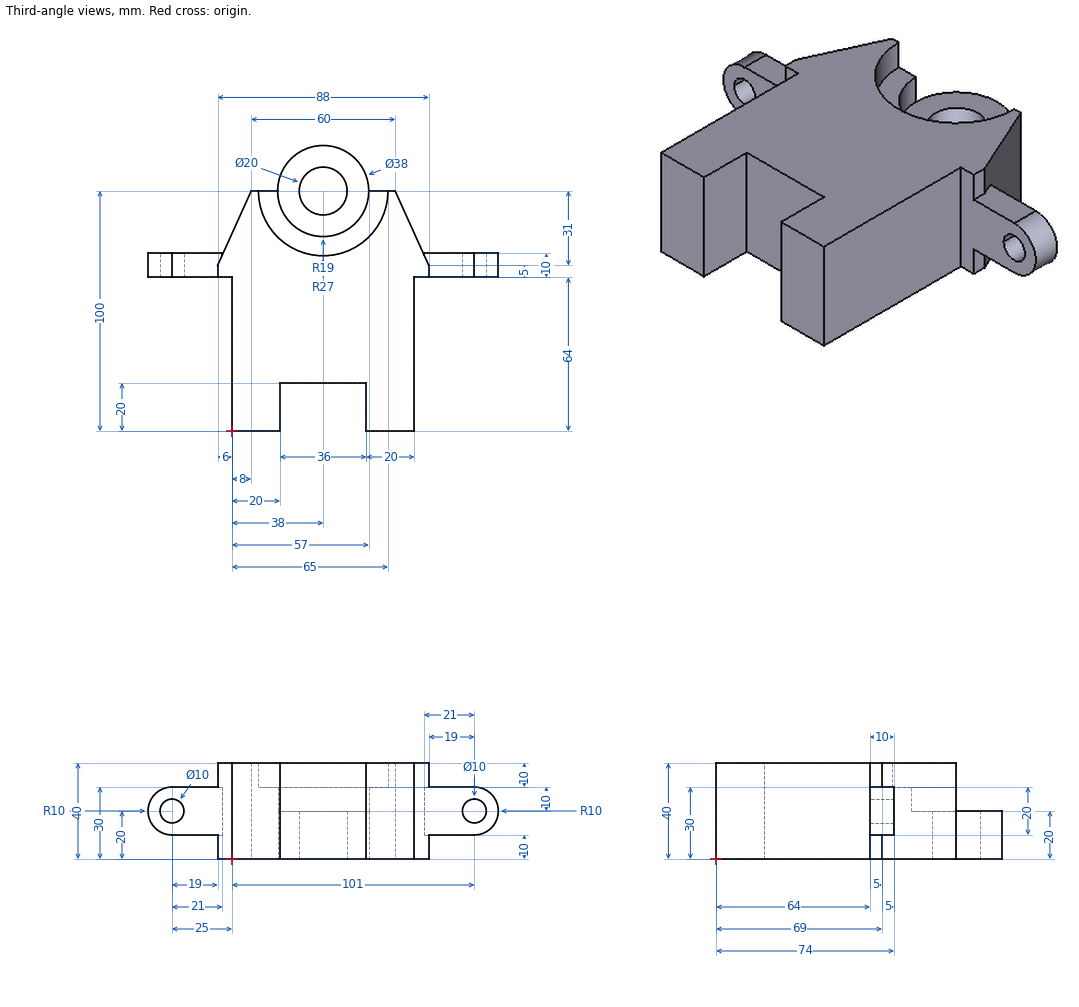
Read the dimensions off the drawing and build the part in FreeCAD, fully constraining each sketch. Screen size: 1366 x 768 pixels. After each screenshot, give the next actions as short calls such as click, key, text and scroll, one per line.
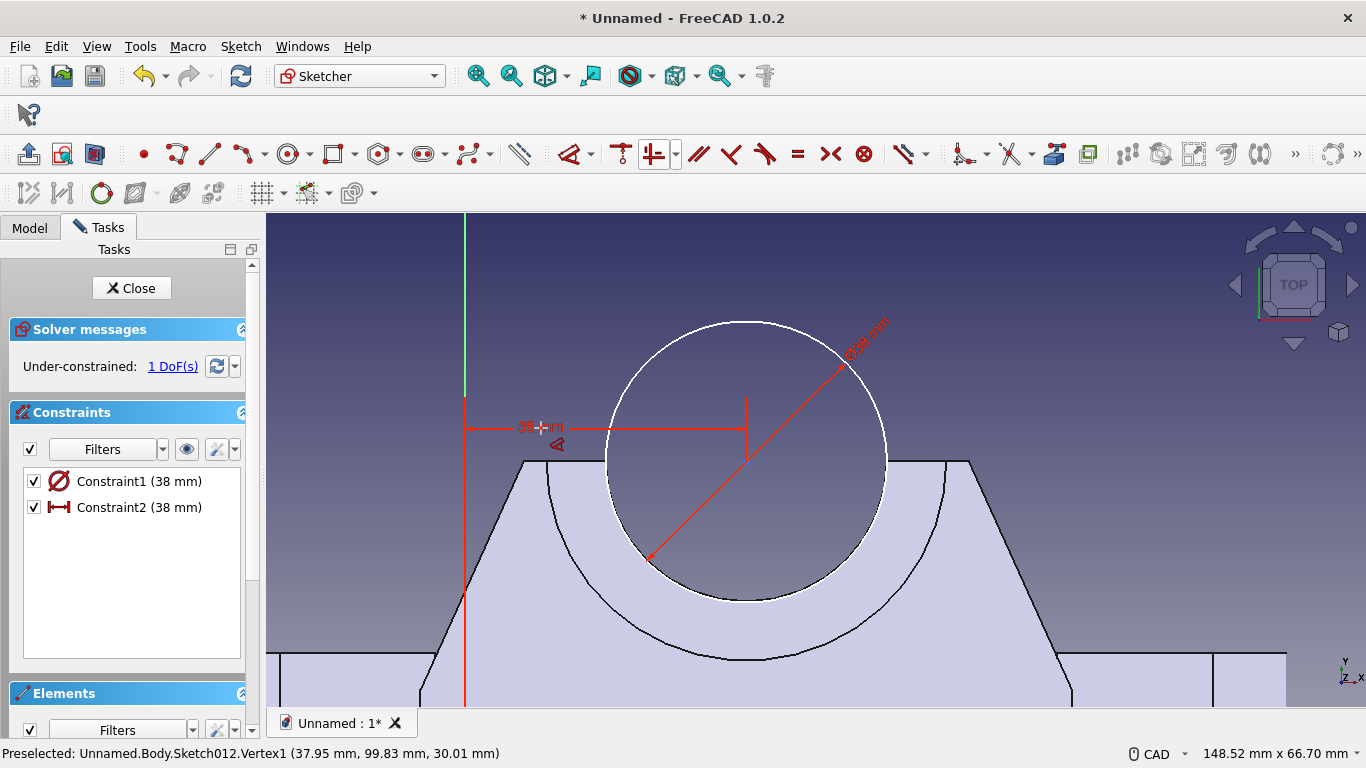
click(746, 462)
click(431, 571)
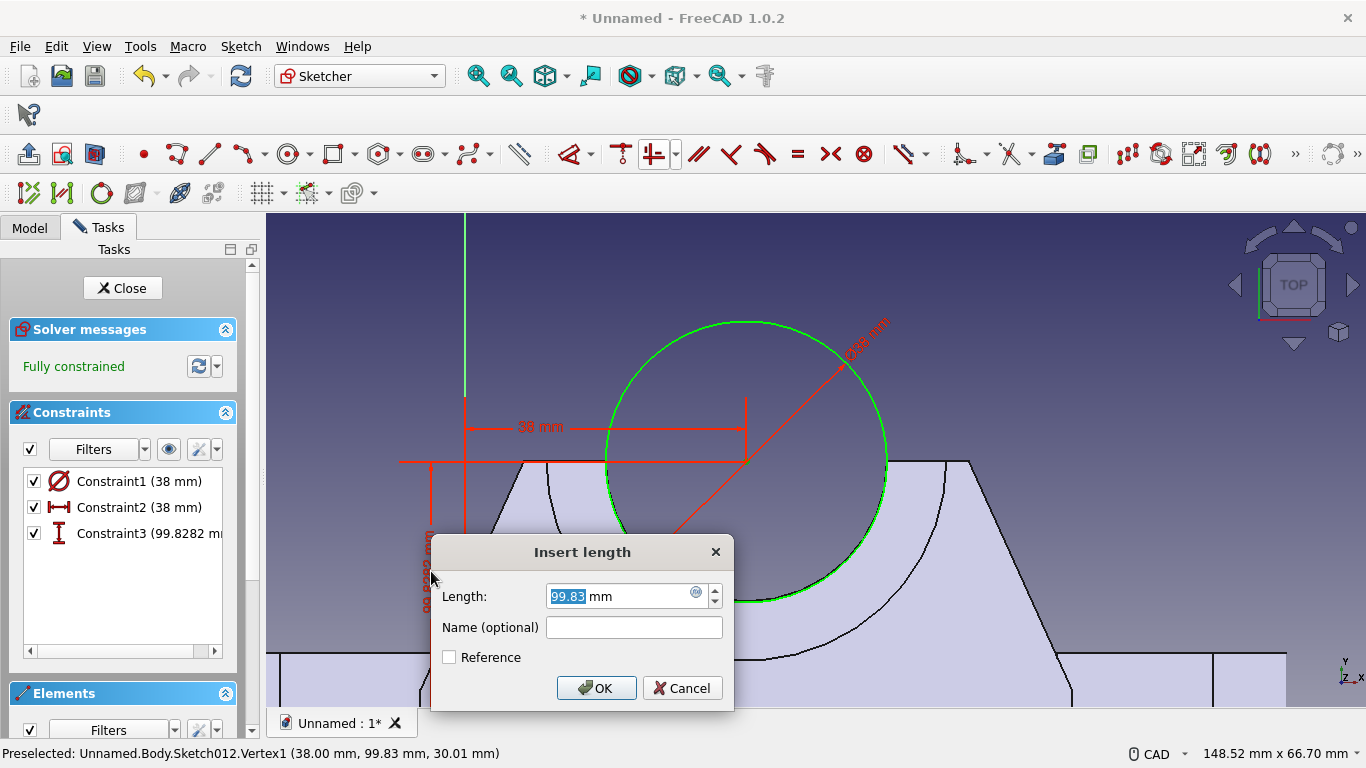
text(100)
key(Return)
key(Escape)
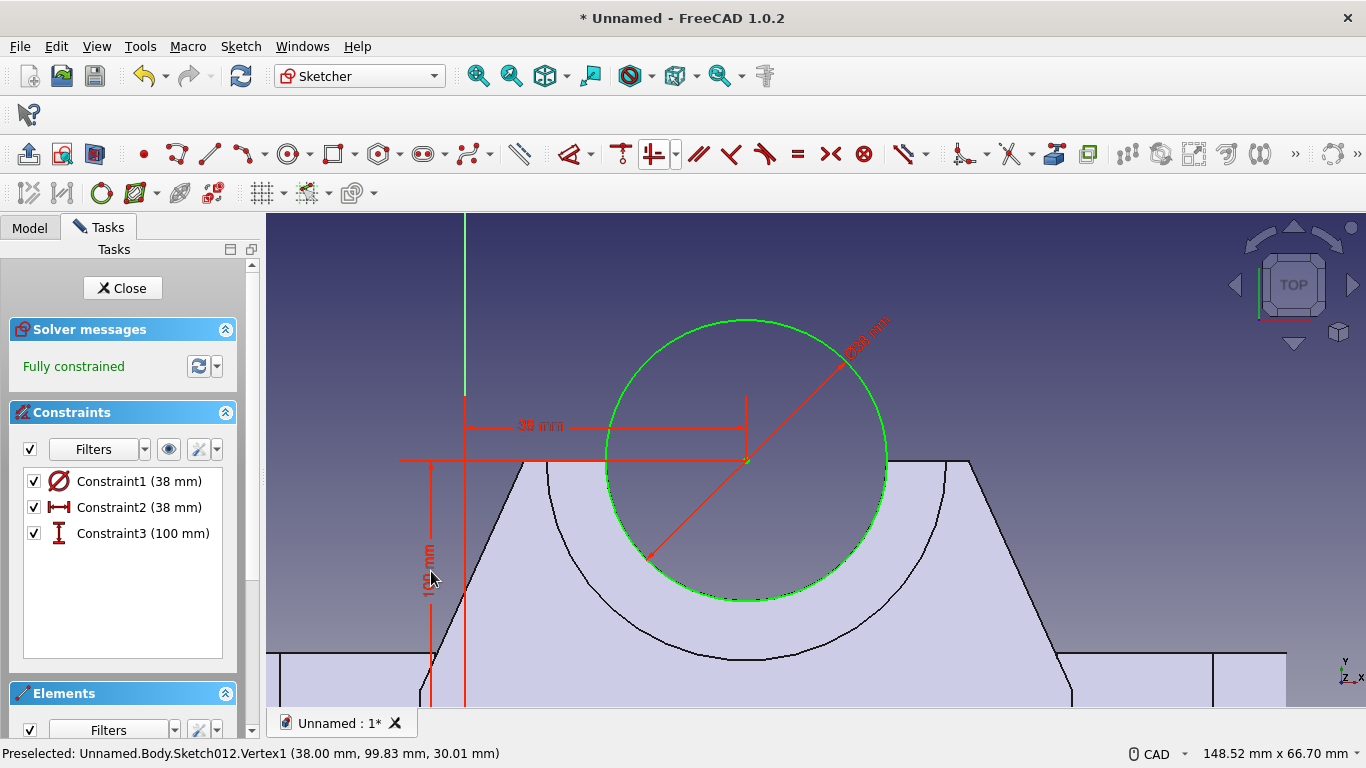
click(123, 288)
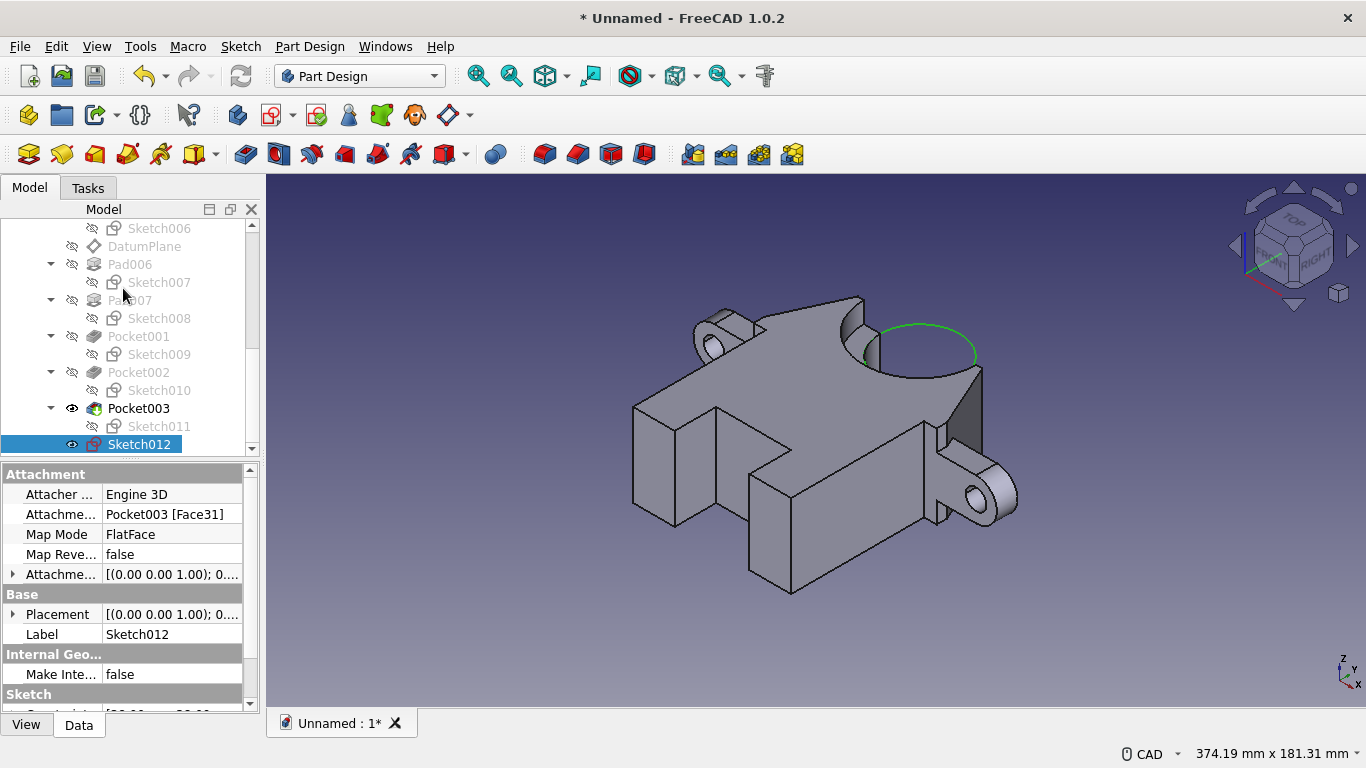
click(29, 154)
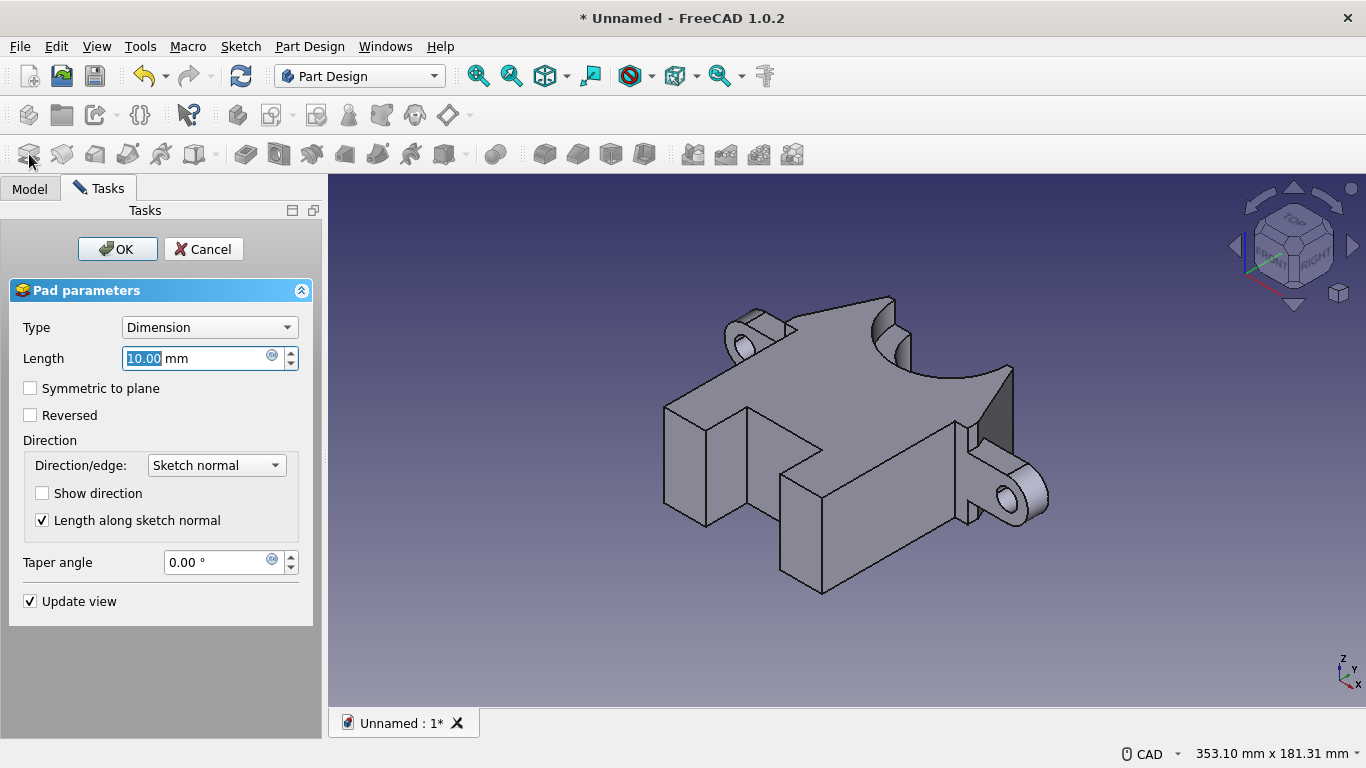
text(30)
key(Tab)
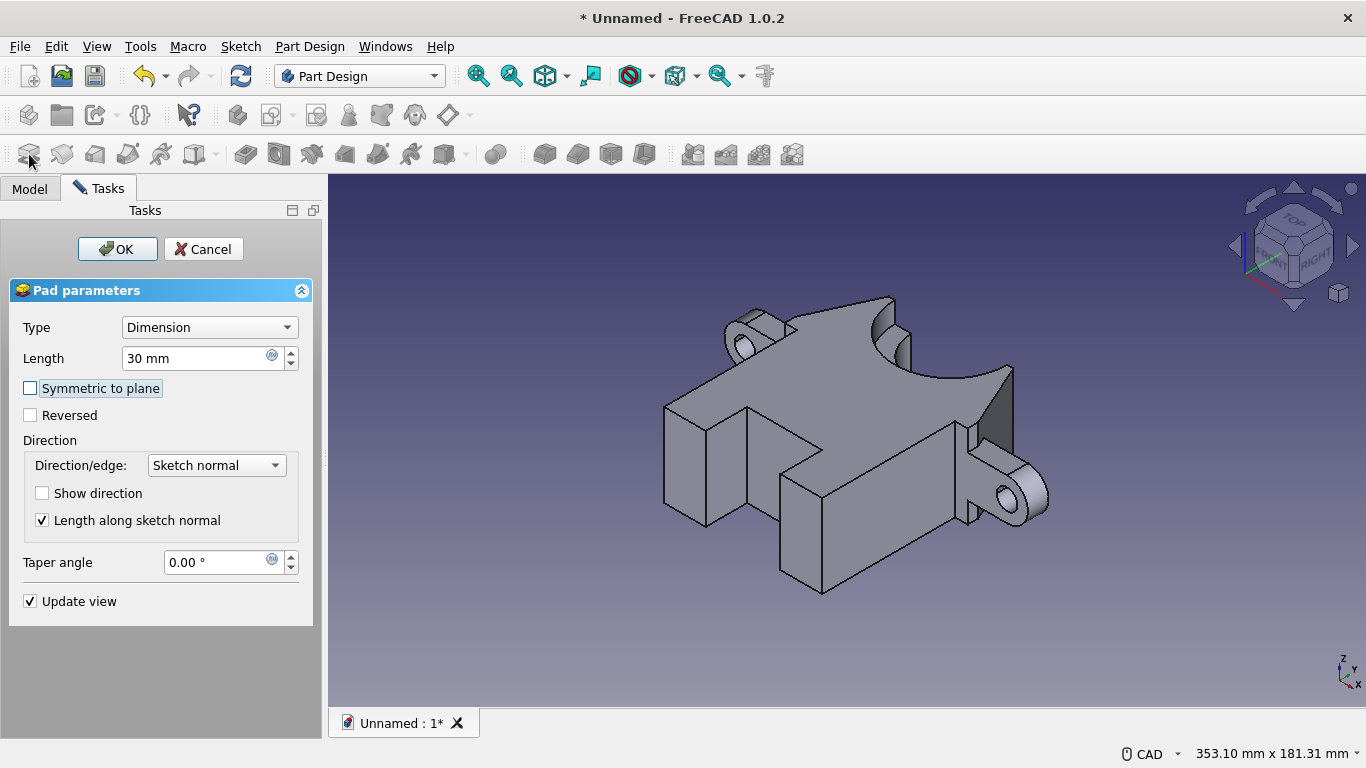
click(31, 415)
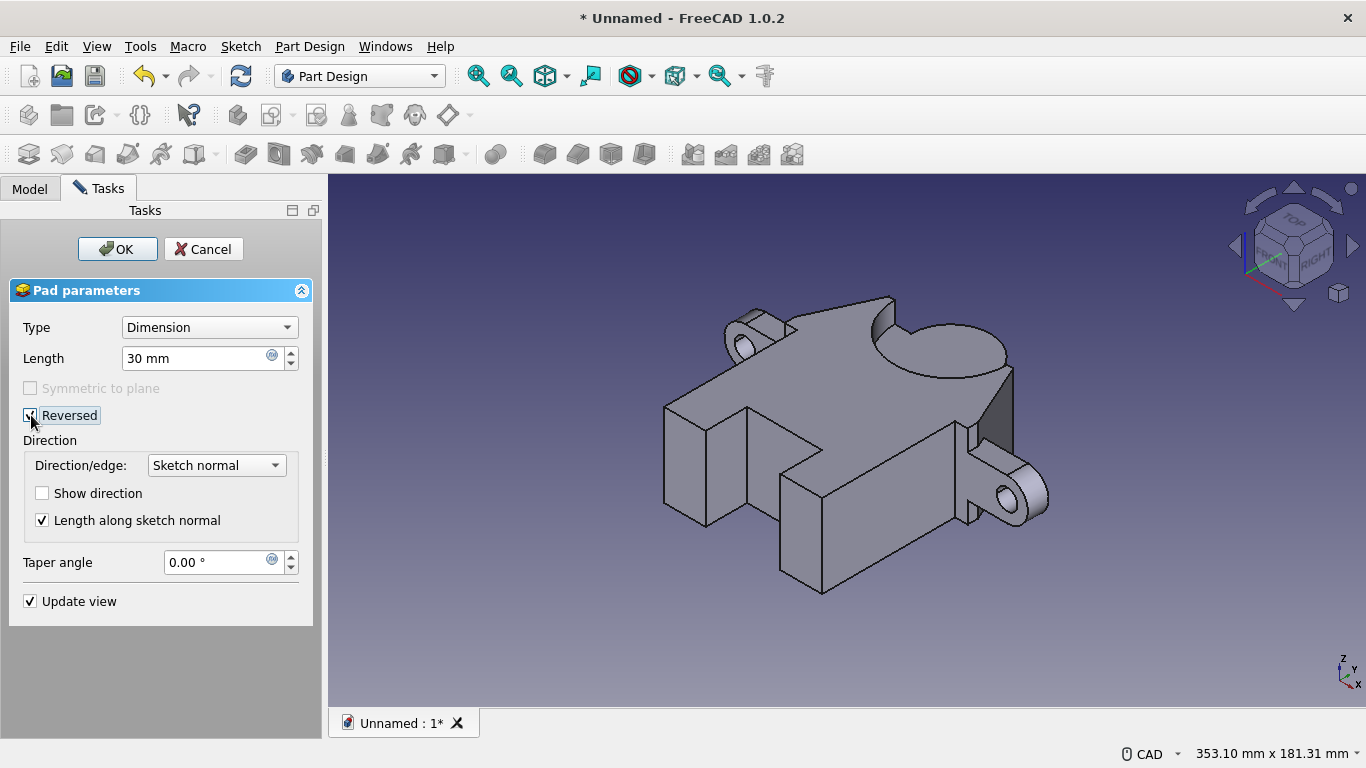
click(118, 249)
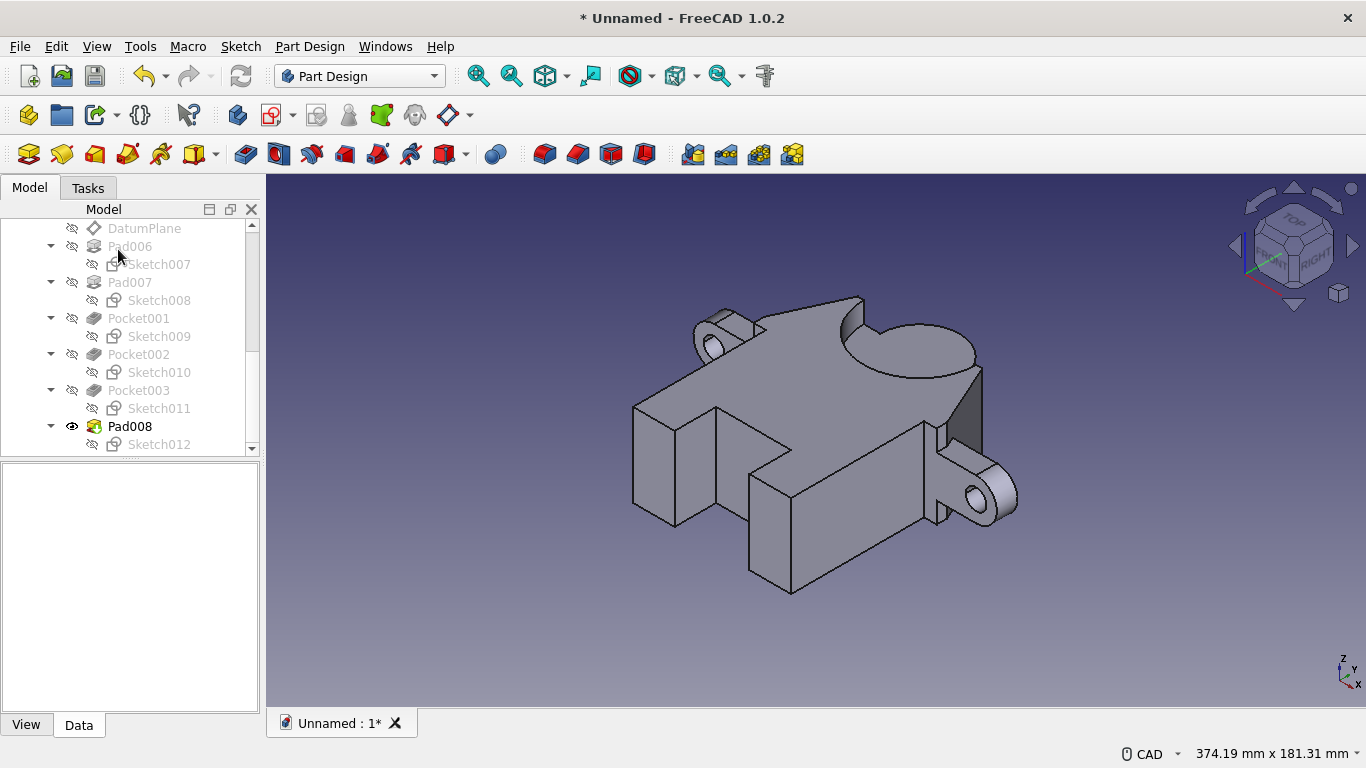
click(912, 360)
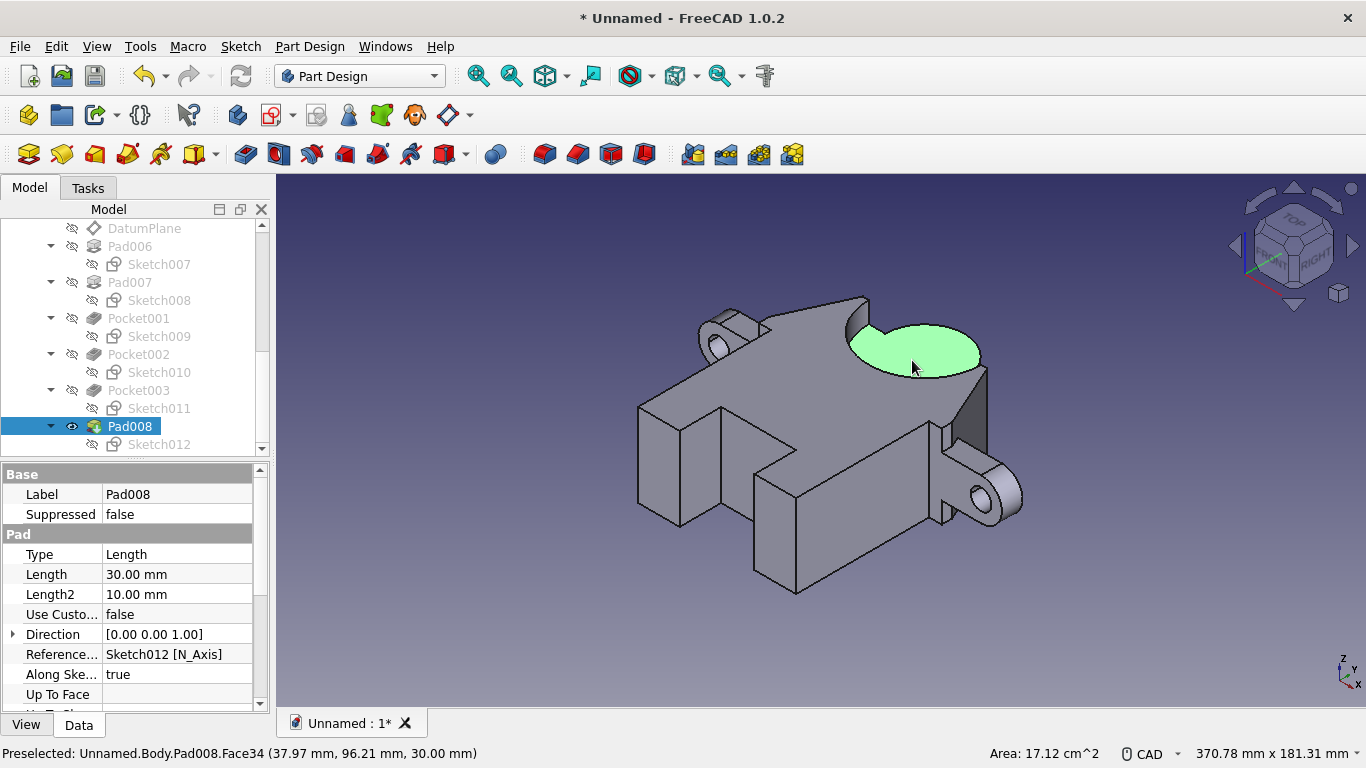
click(270, 116)